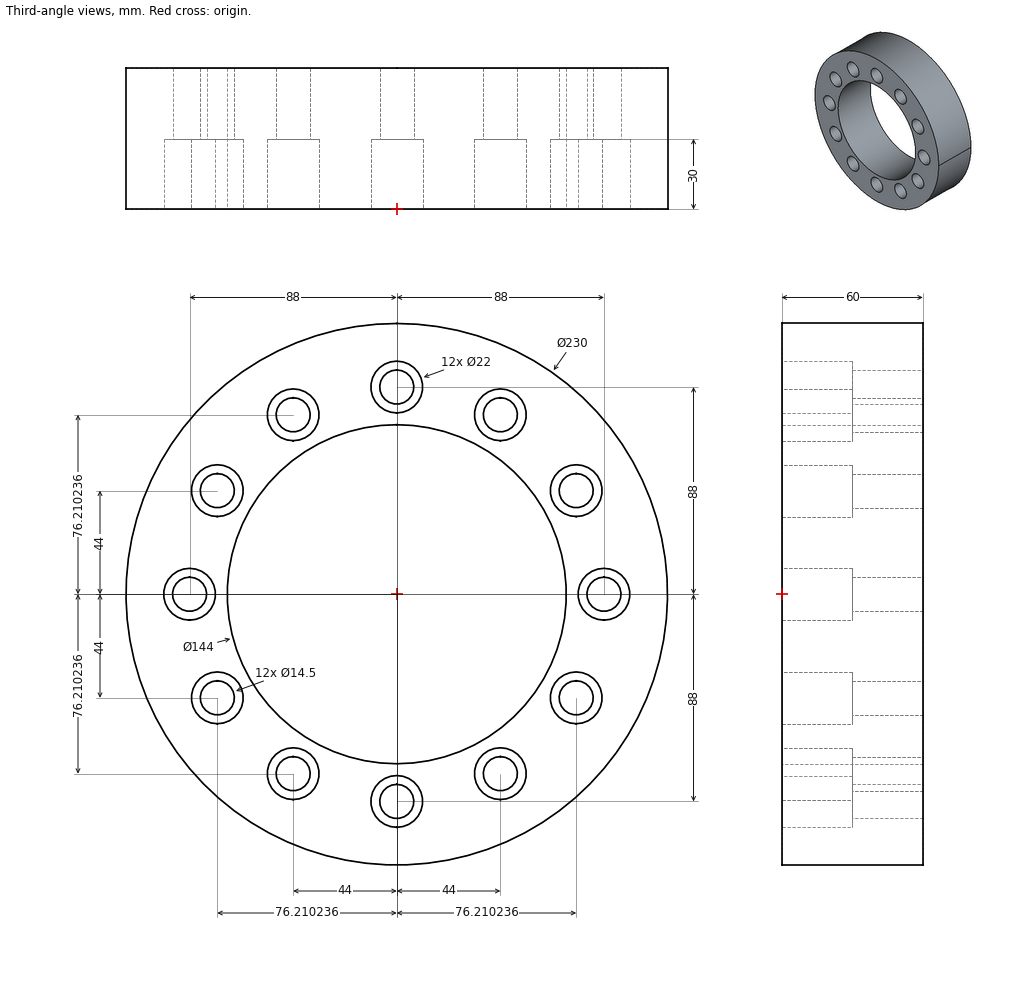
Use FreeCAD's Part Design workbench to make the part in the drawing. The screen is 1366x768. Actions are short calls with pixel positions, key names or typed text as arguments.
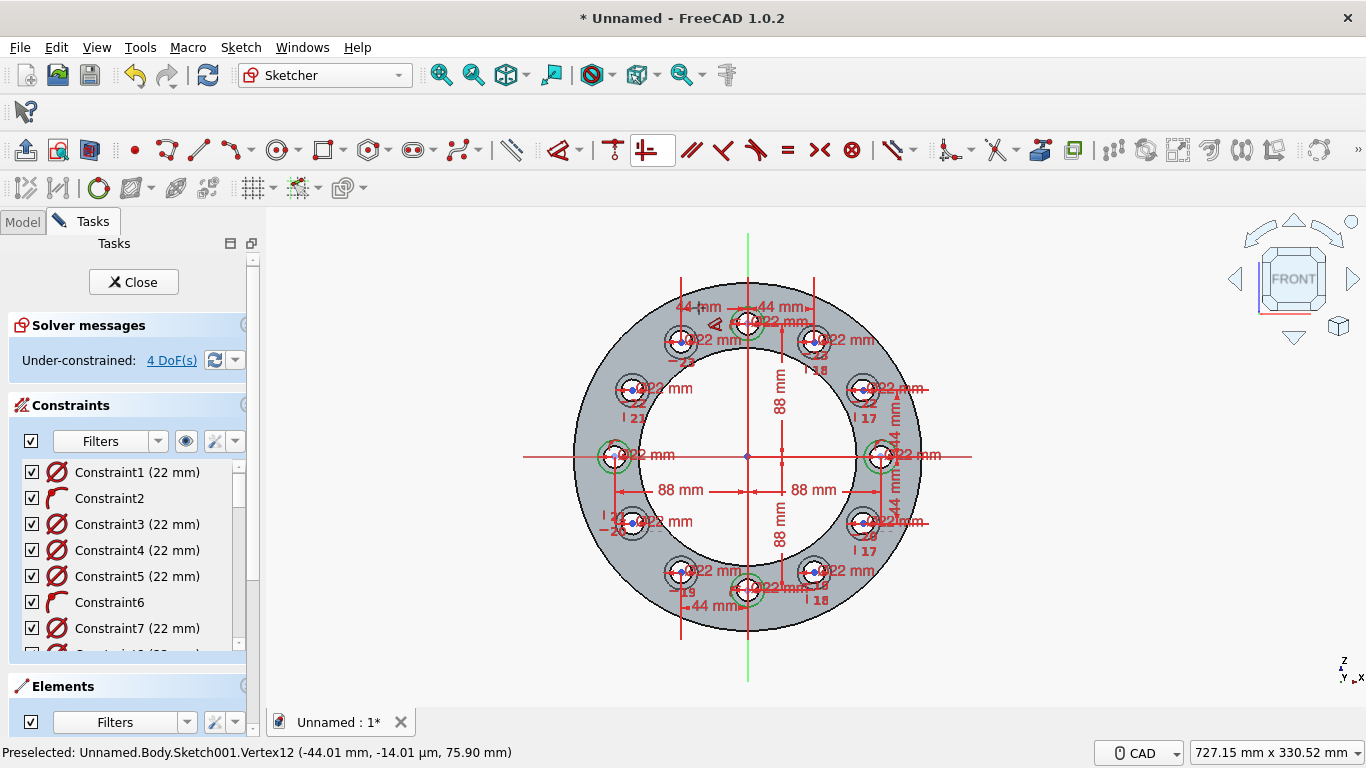
click(814, 342)
click(848, 359)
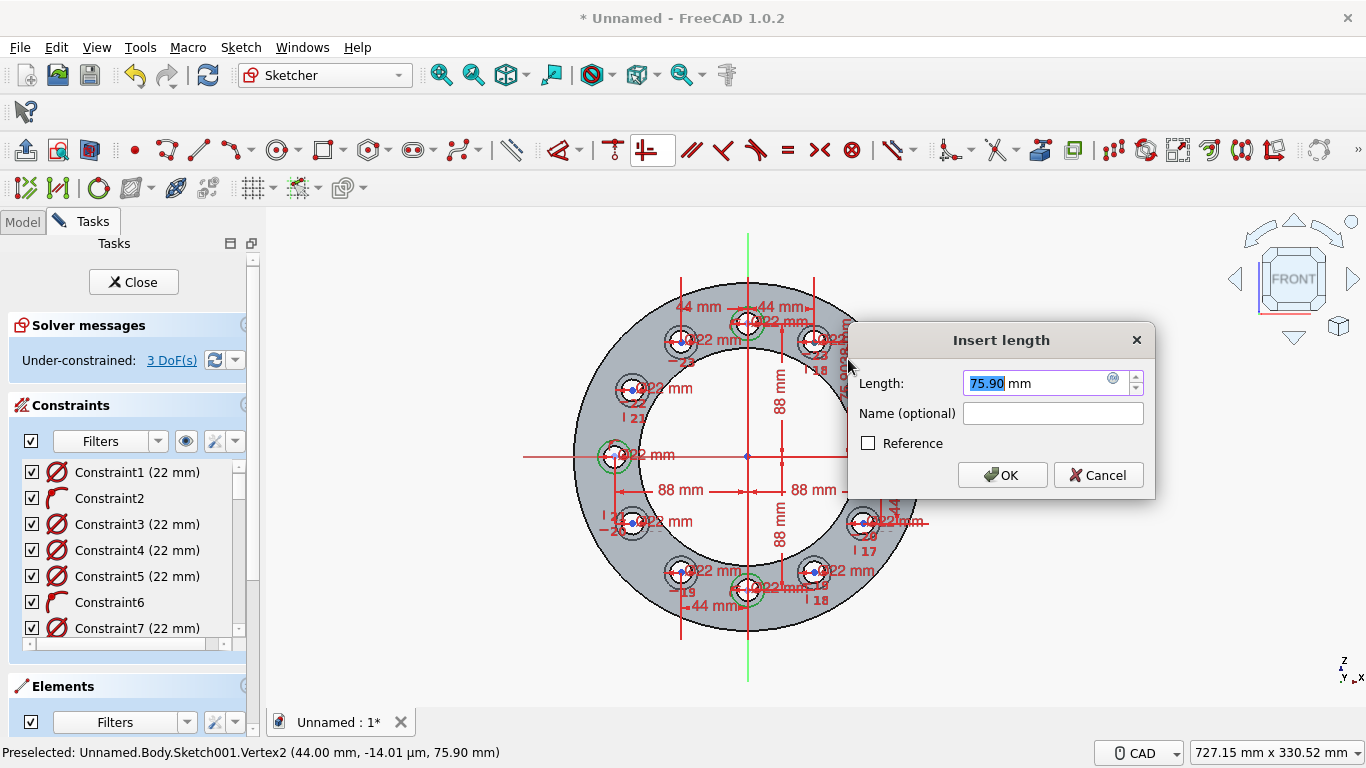
text(76.210236)
key(Return)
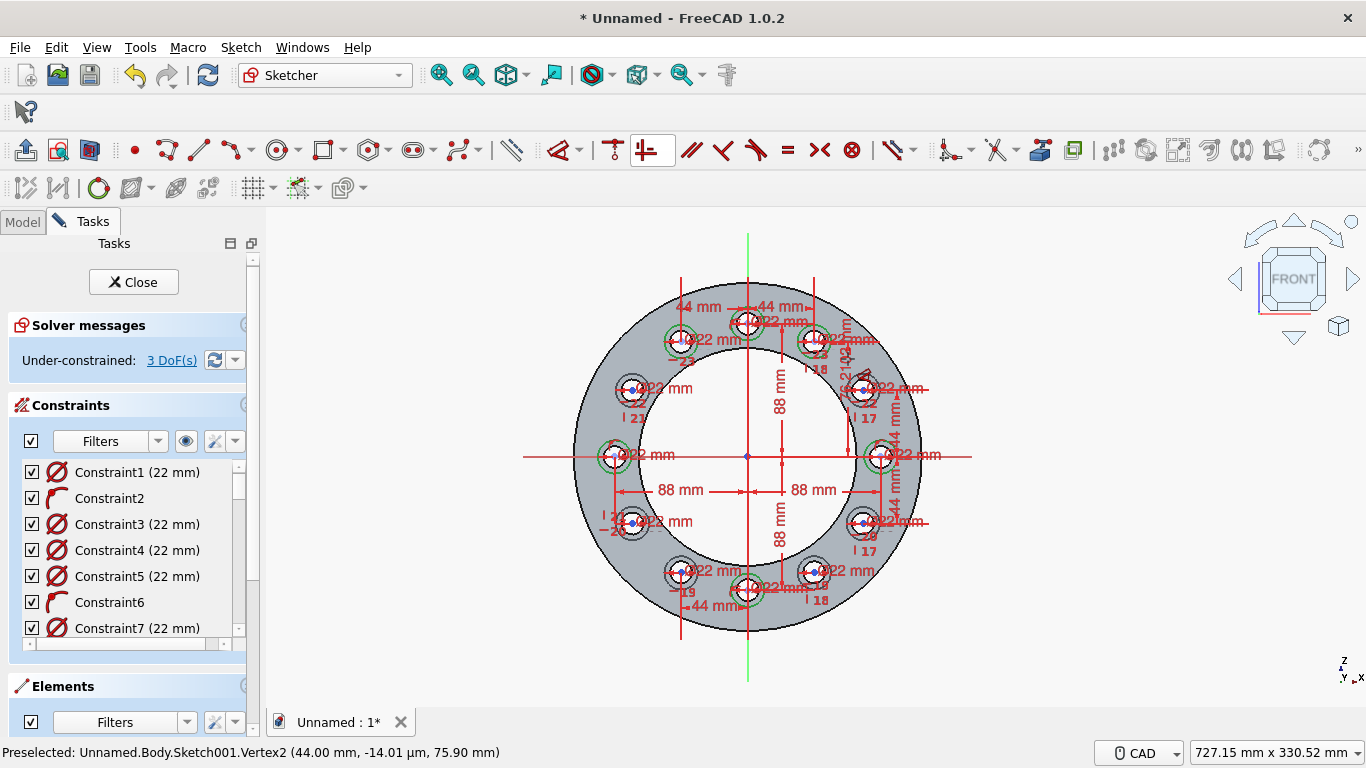
click(863, 390)
click(765, 356)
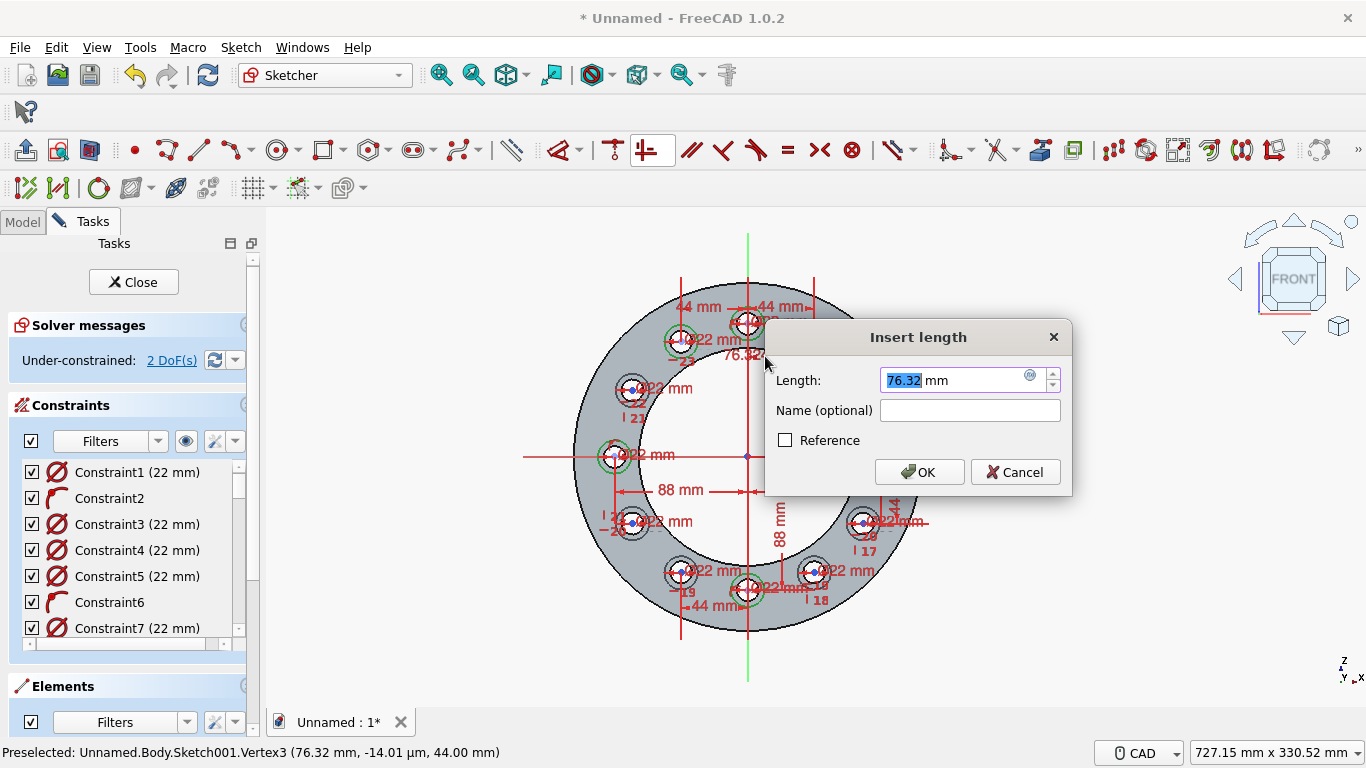
text(76.210236)
key(Return)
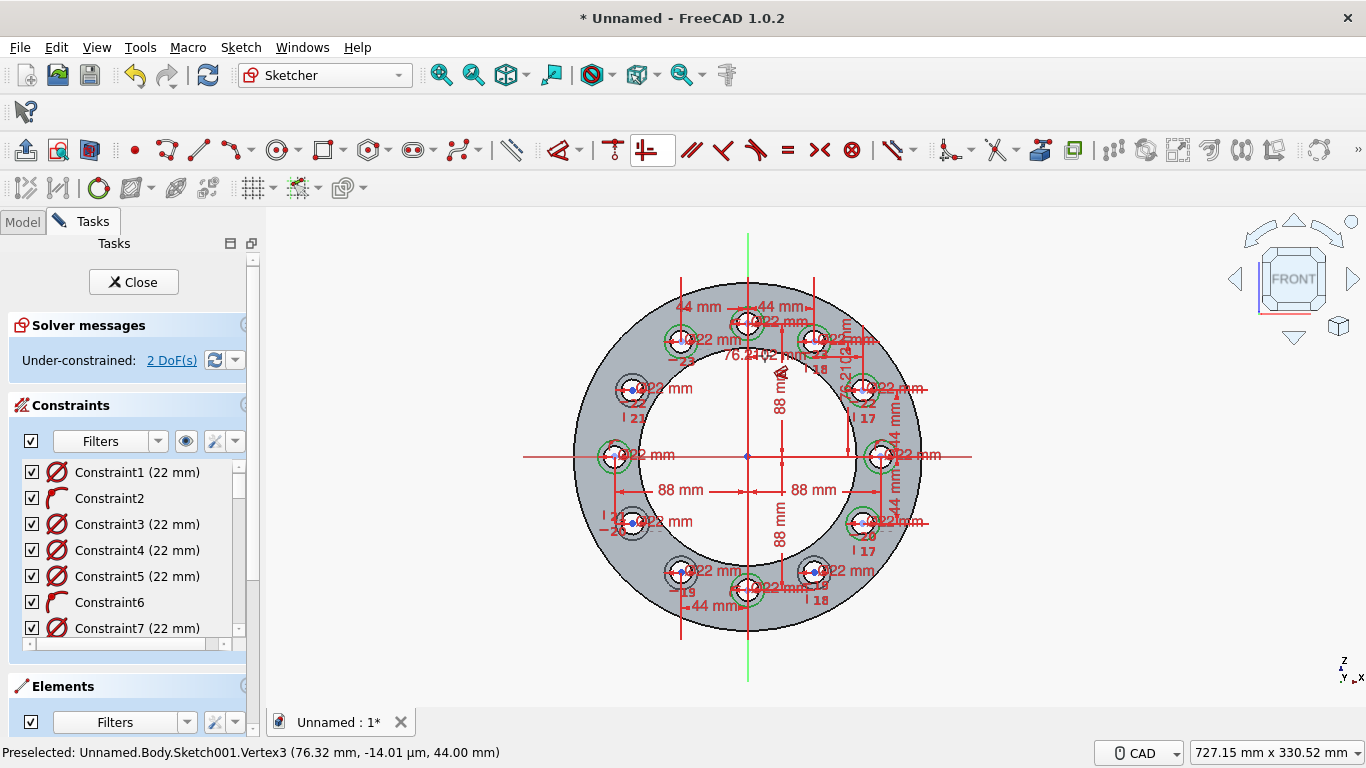
click(814, 573)
click(848, 556)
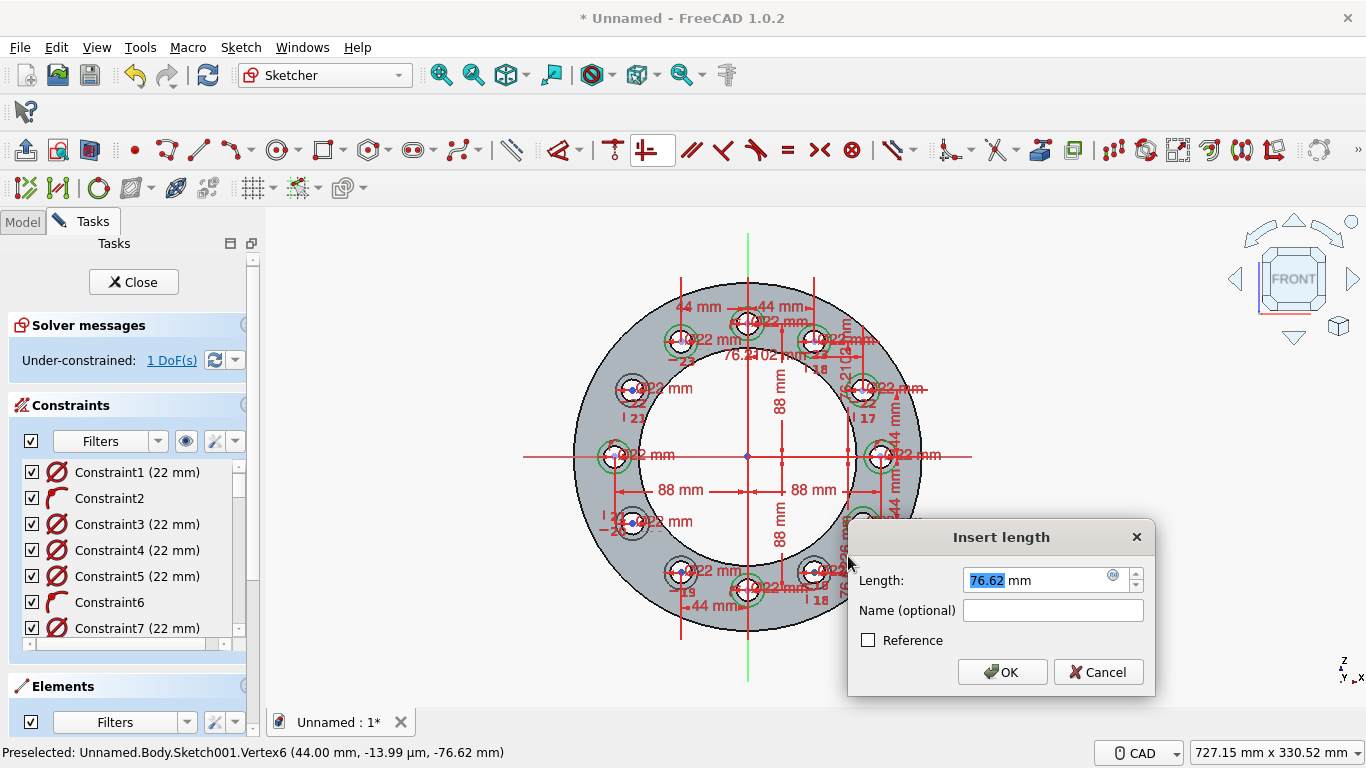
text(76.210236)
key(Return)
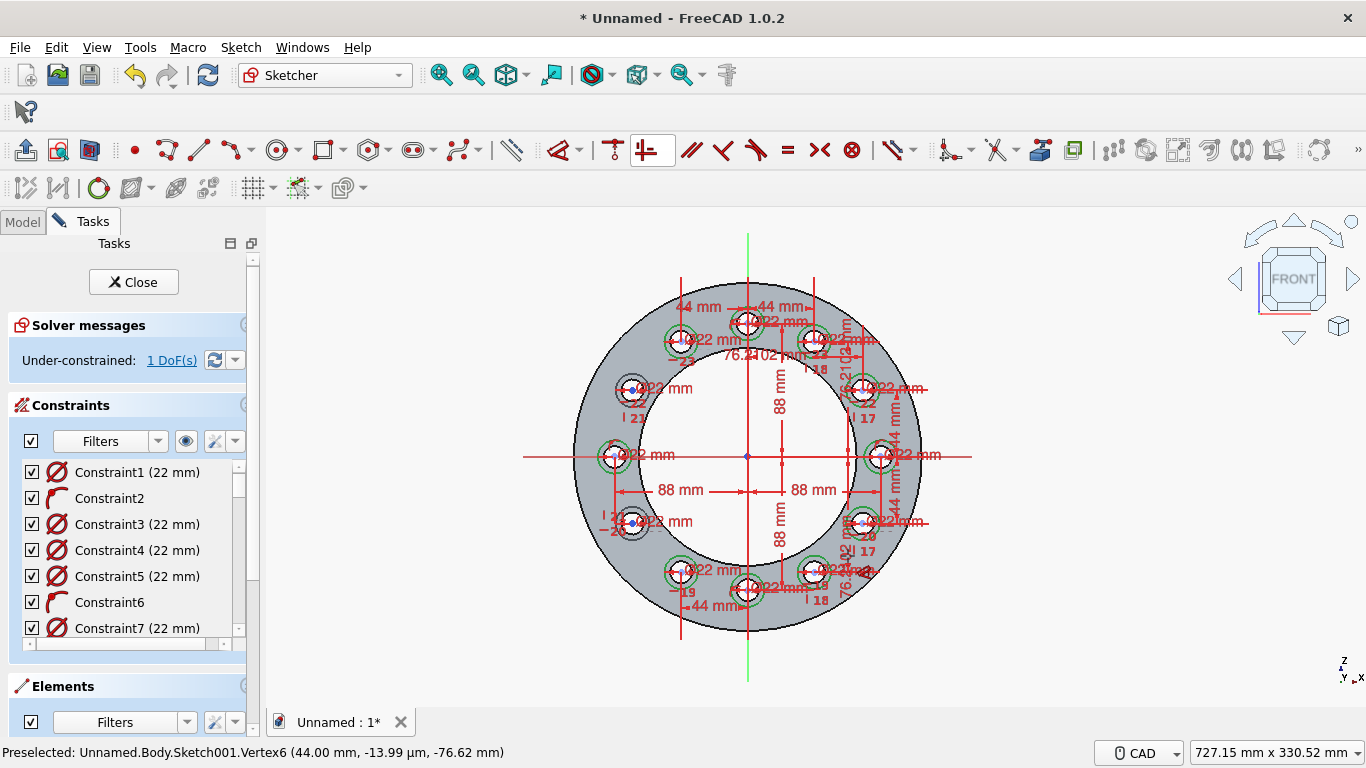
click(633, 524)
click(717, 558)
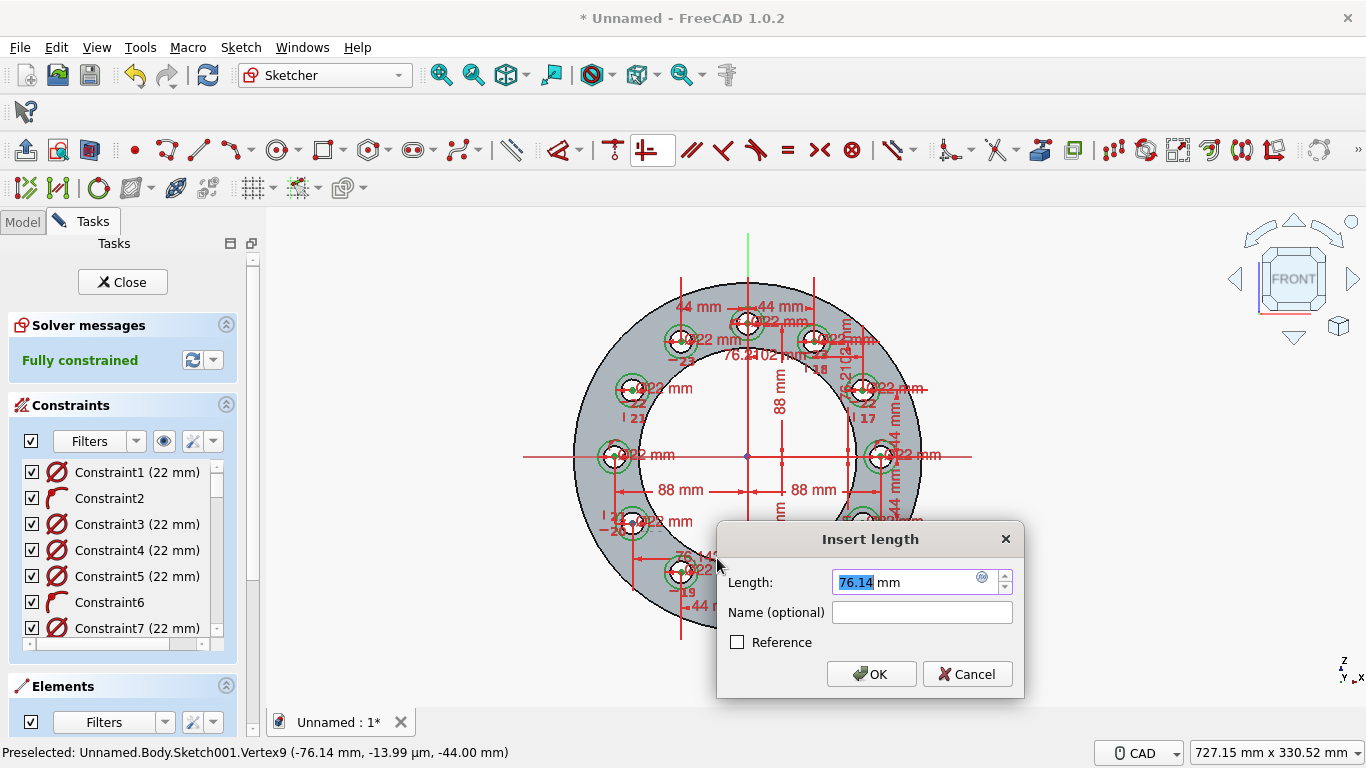
text(76.210236)
key(Return)
key(Escape)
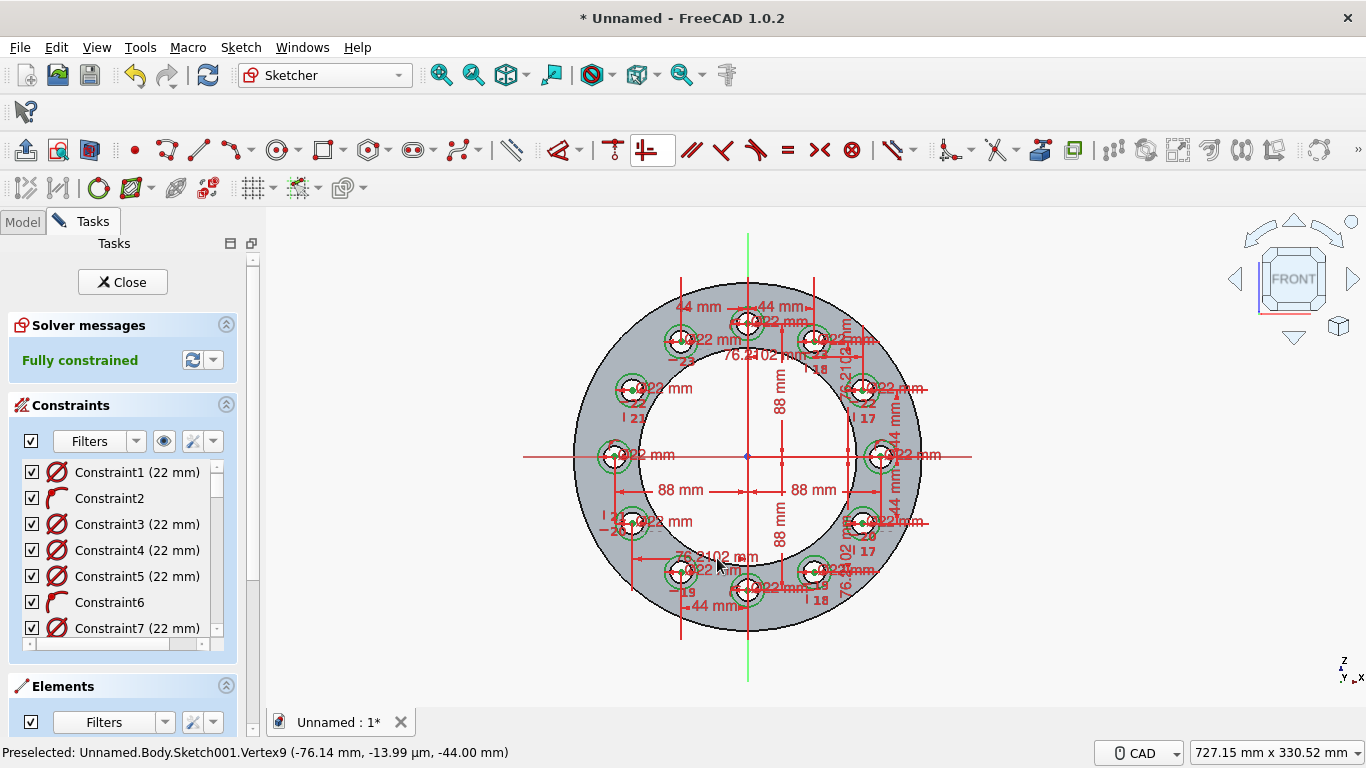
click(123, 282)